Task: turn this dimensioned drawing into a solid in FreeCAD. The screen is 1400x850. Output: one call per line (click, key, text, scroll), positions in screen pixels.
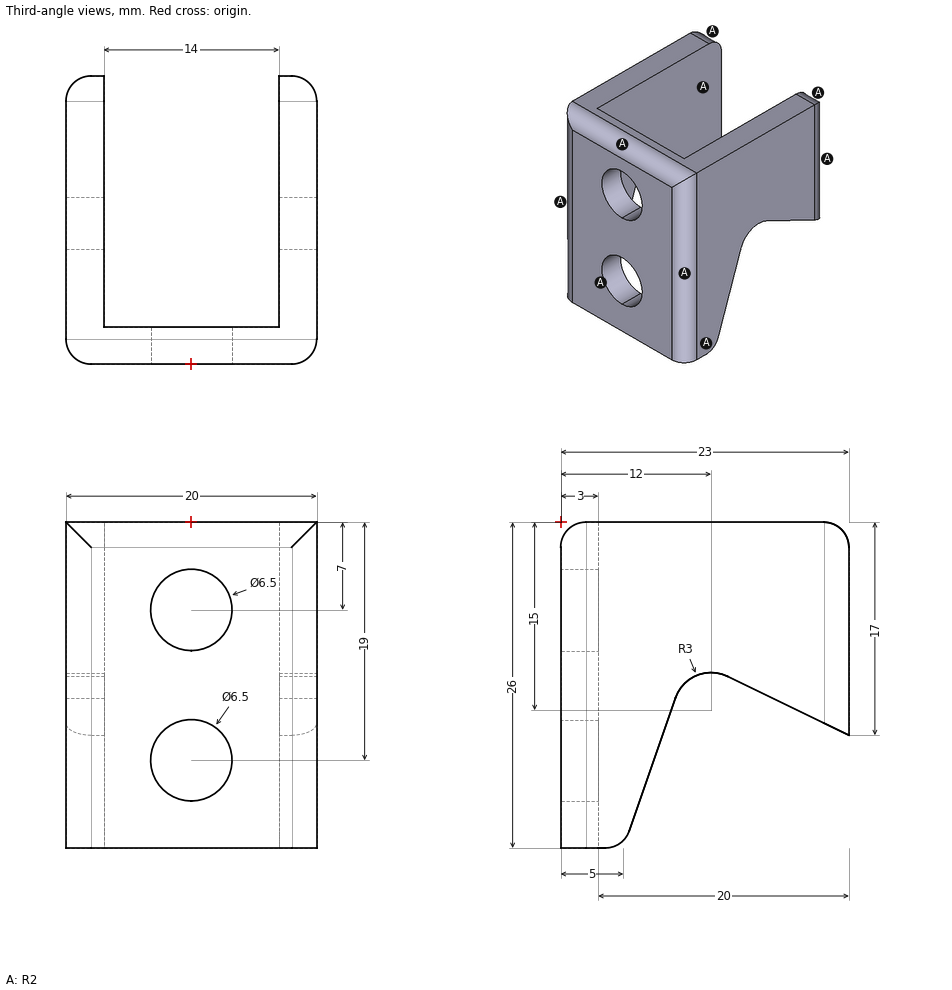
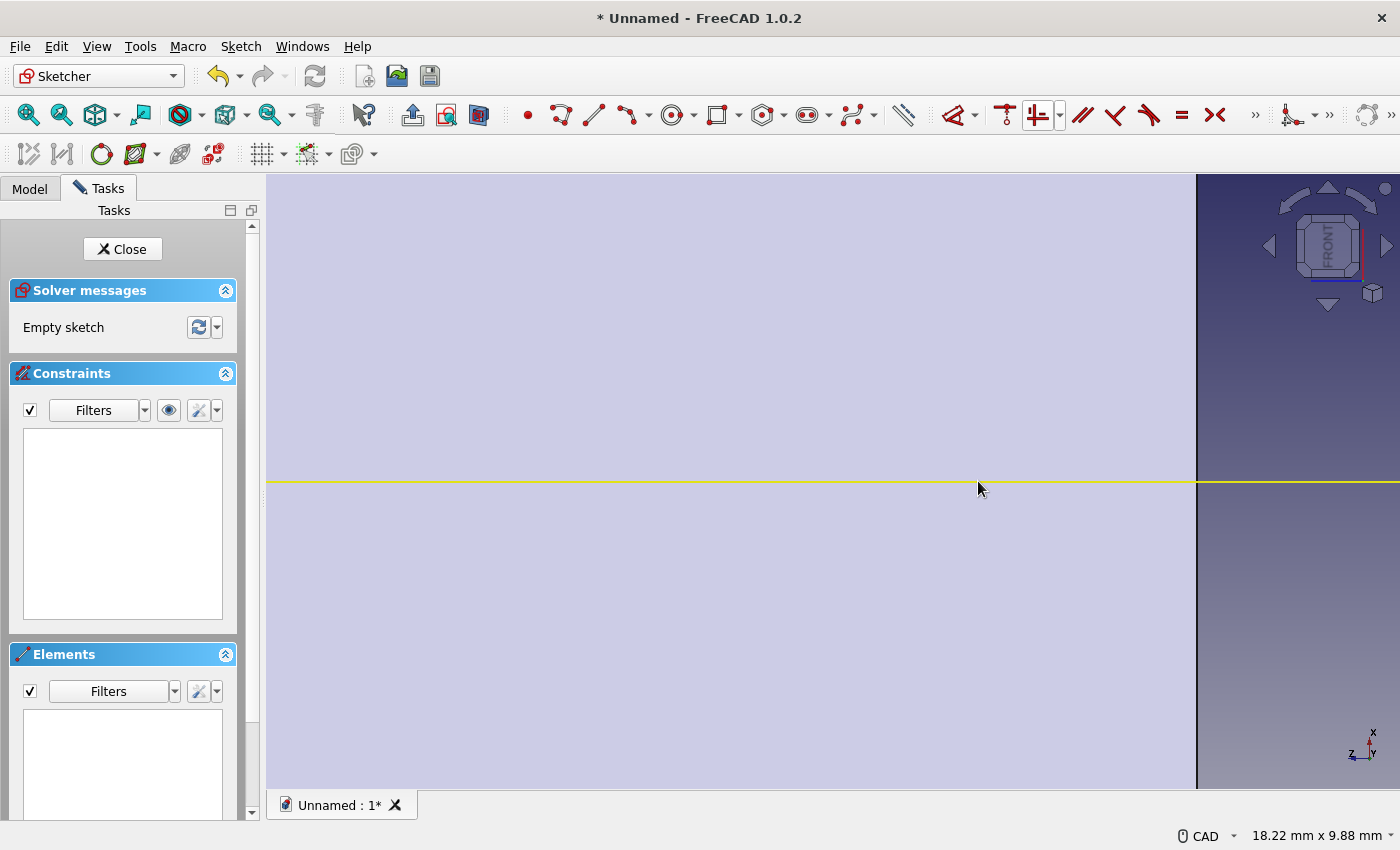
click(672, 116)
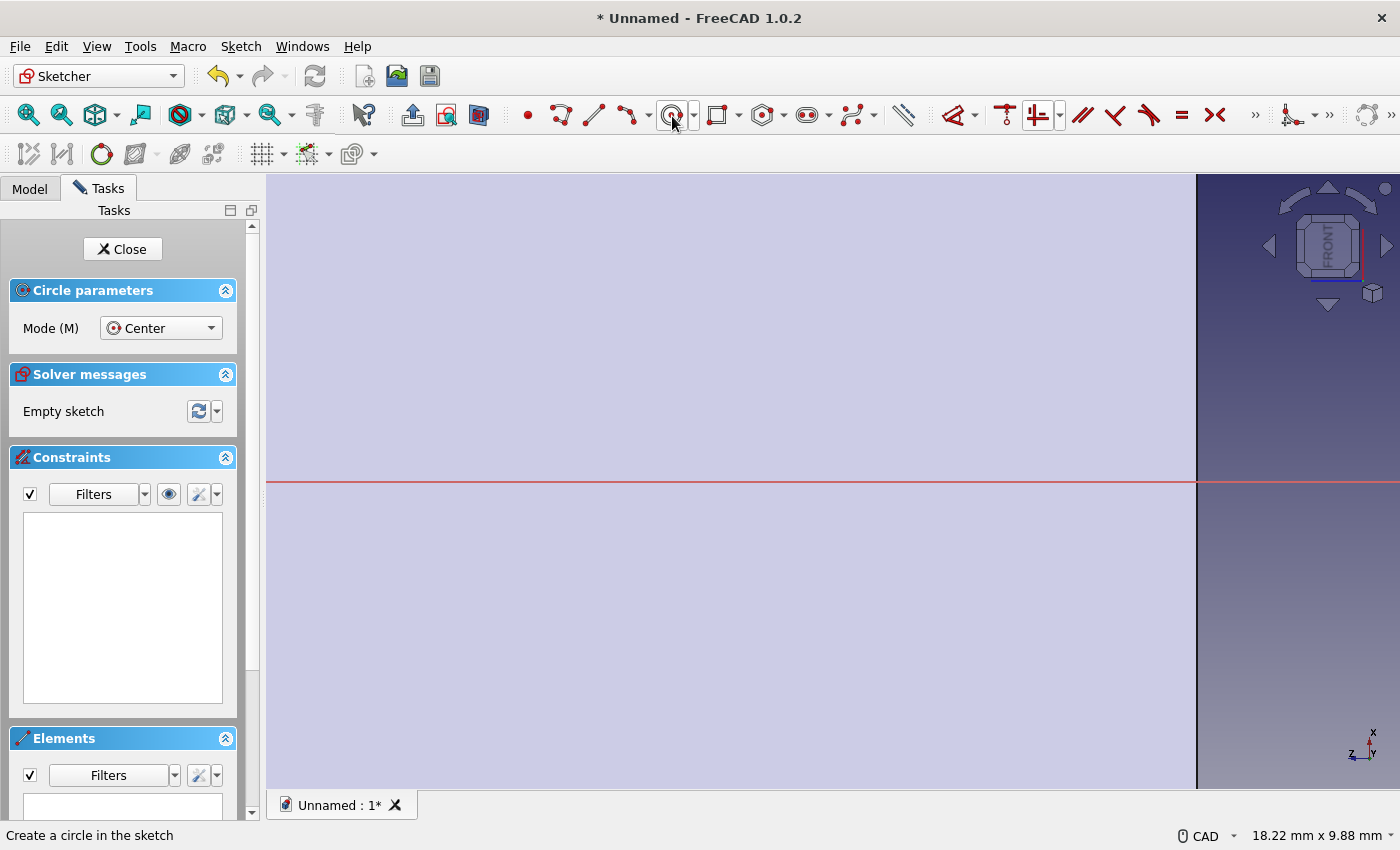
click(762, 482)
click(905, 338)
key(Escape)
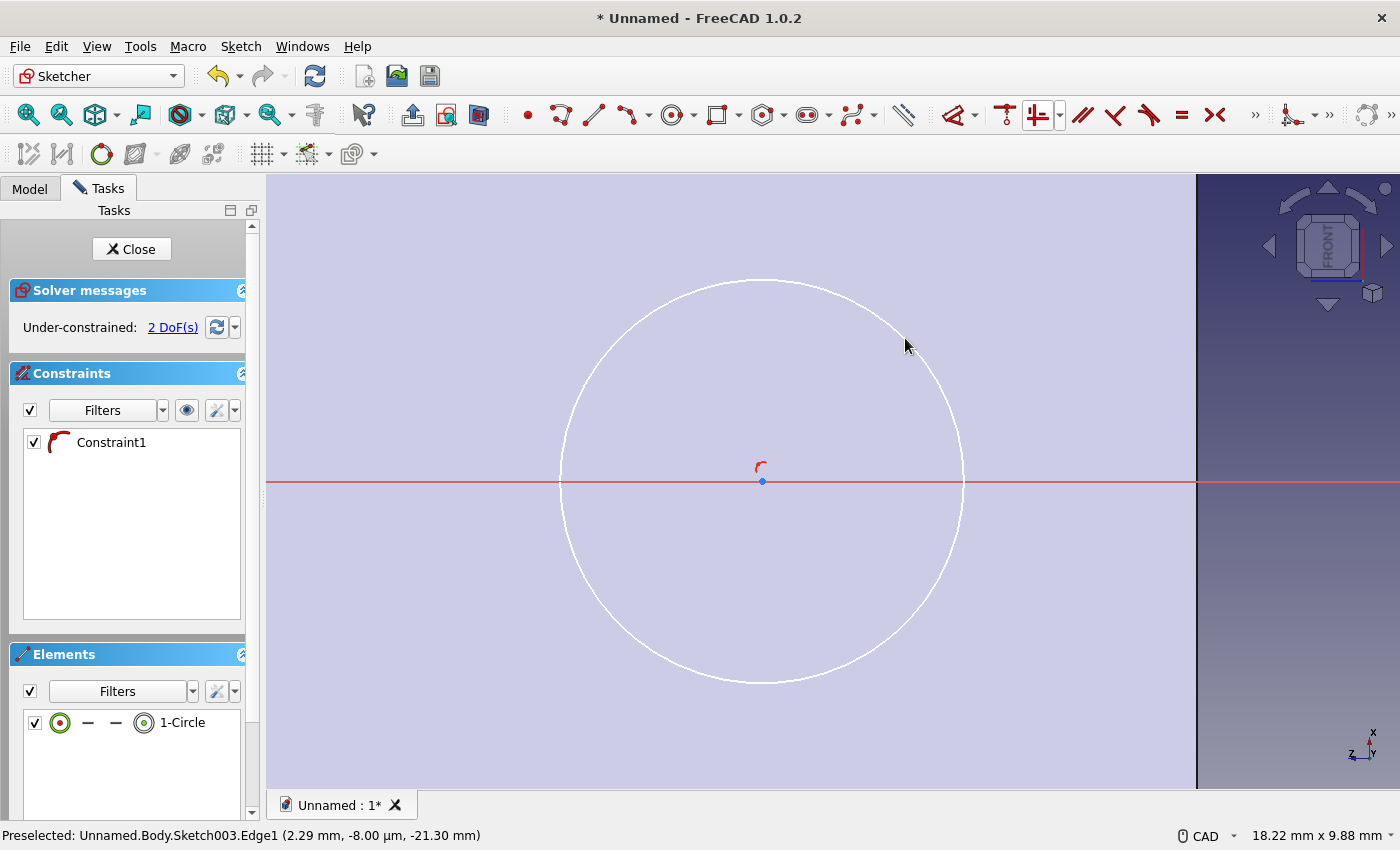
click(952, 116)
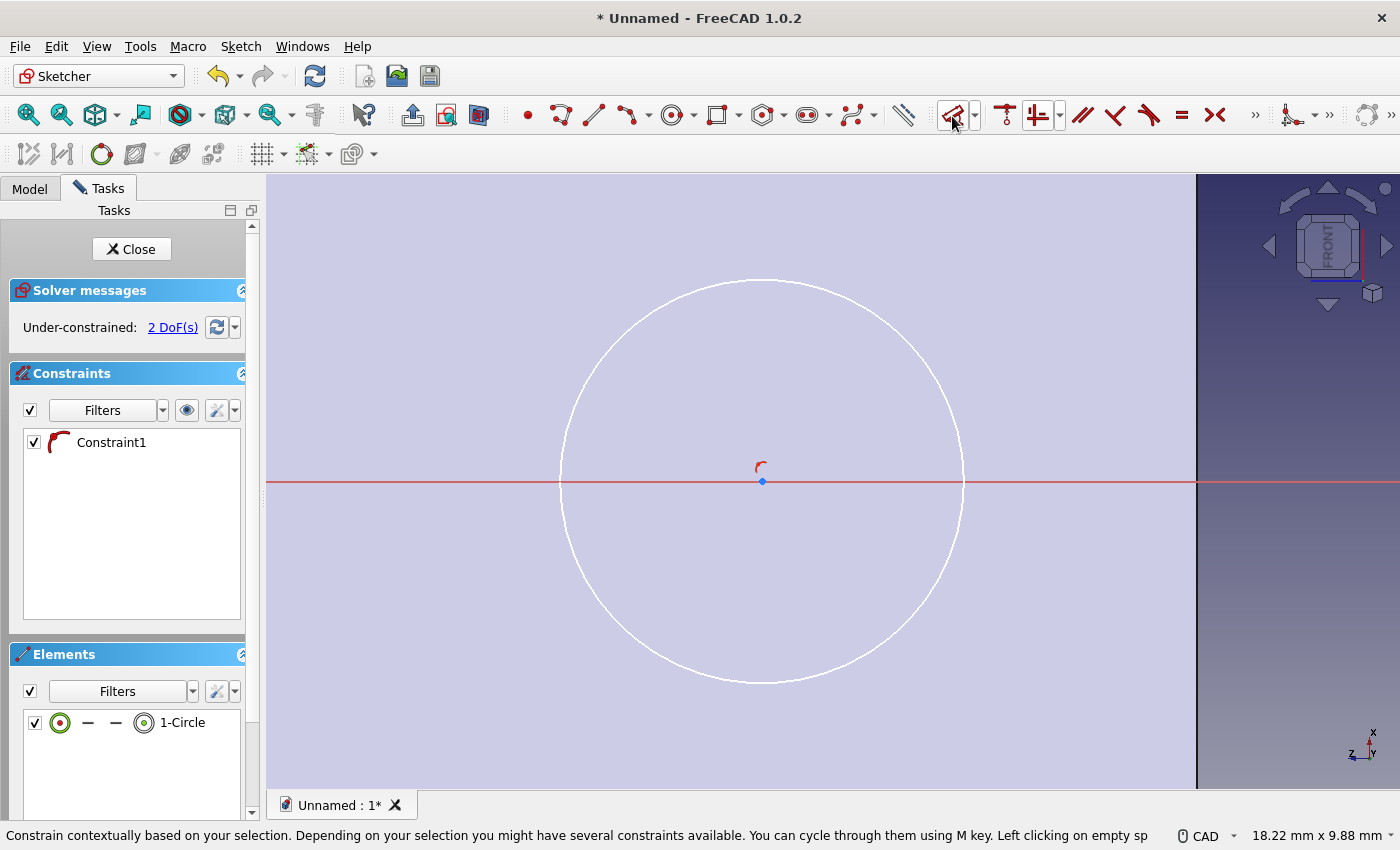
click(904, 338)
click(927, 315)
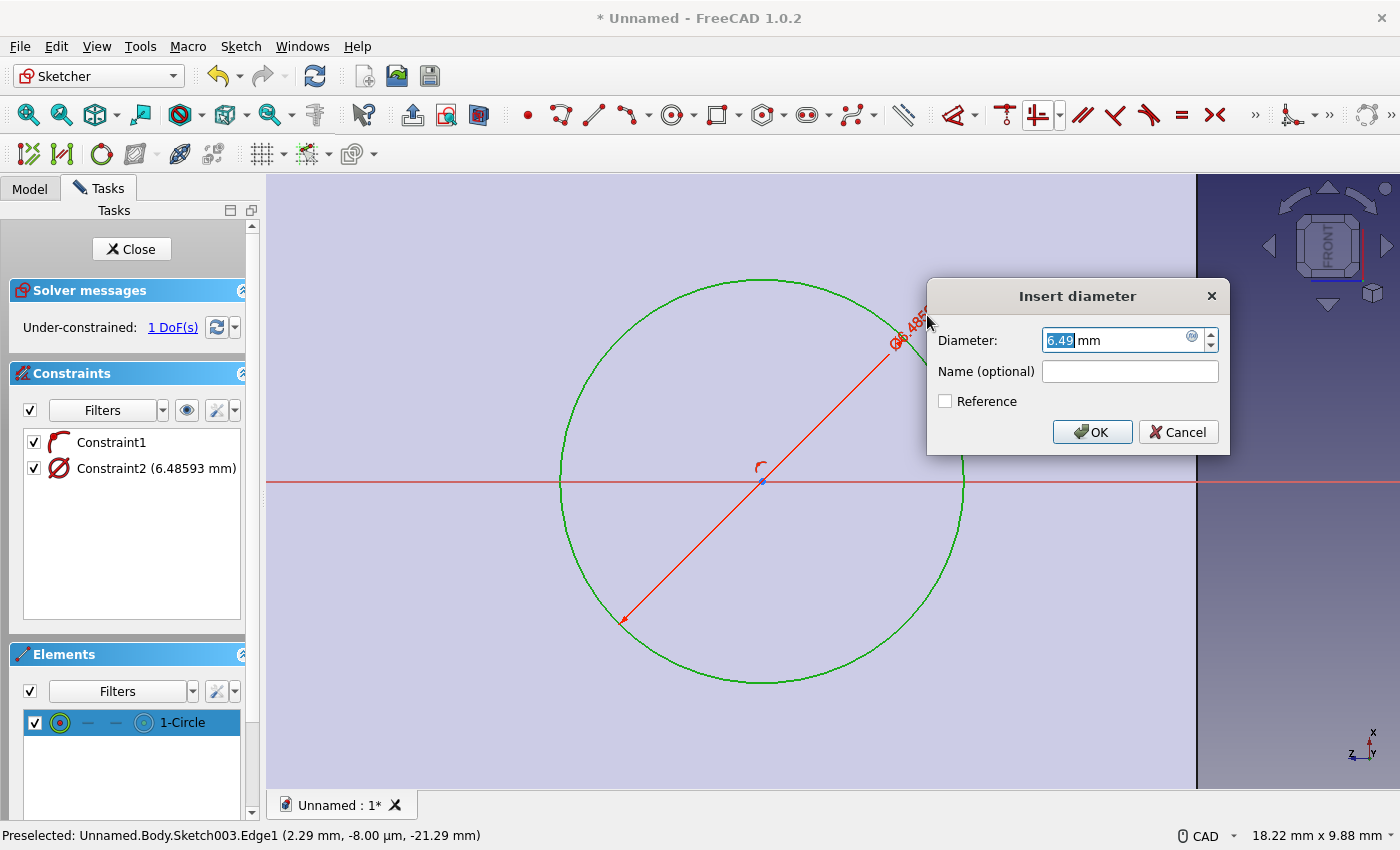
text(6.5)
key(Return)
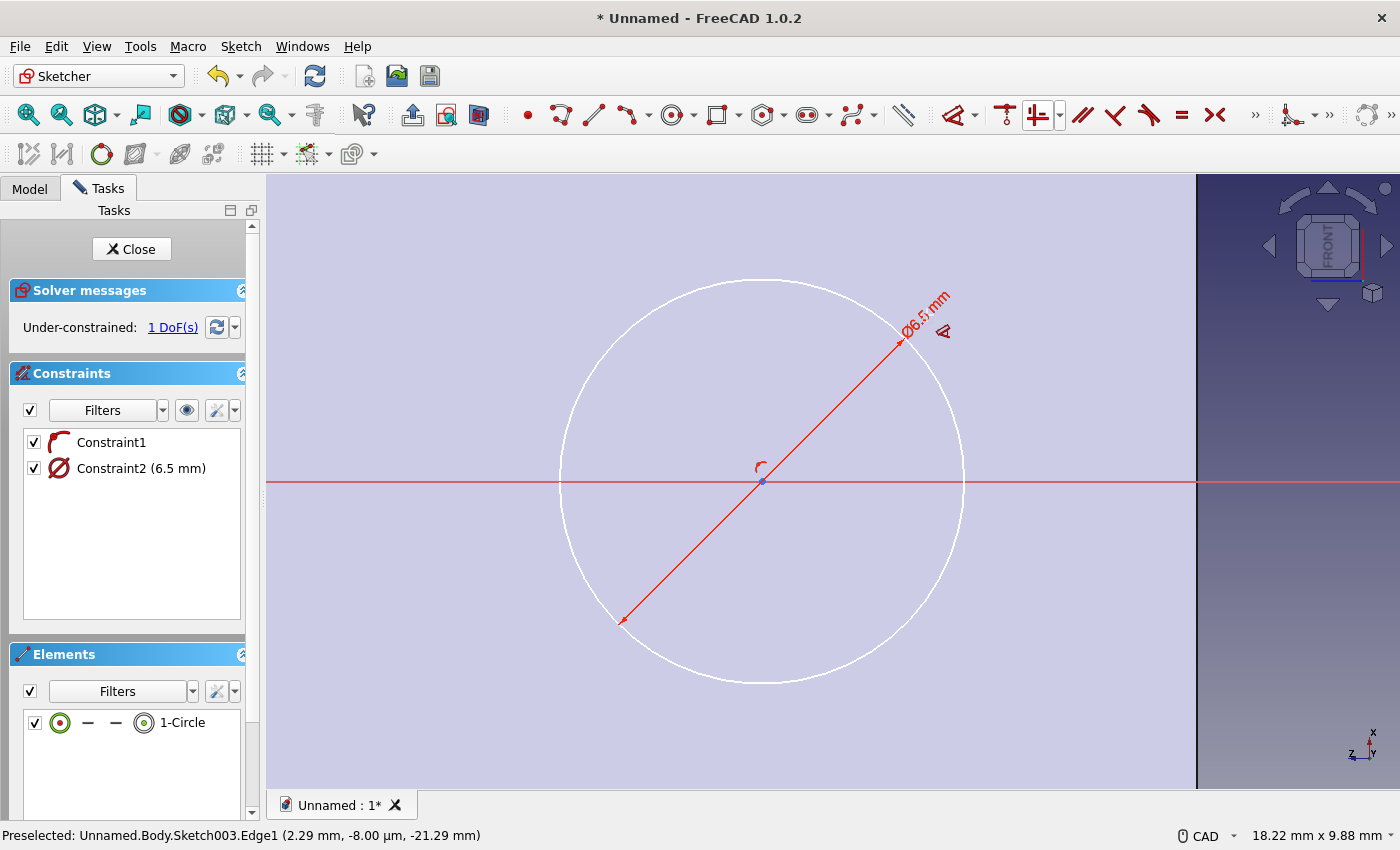
click(762, 482)
click(528, 516)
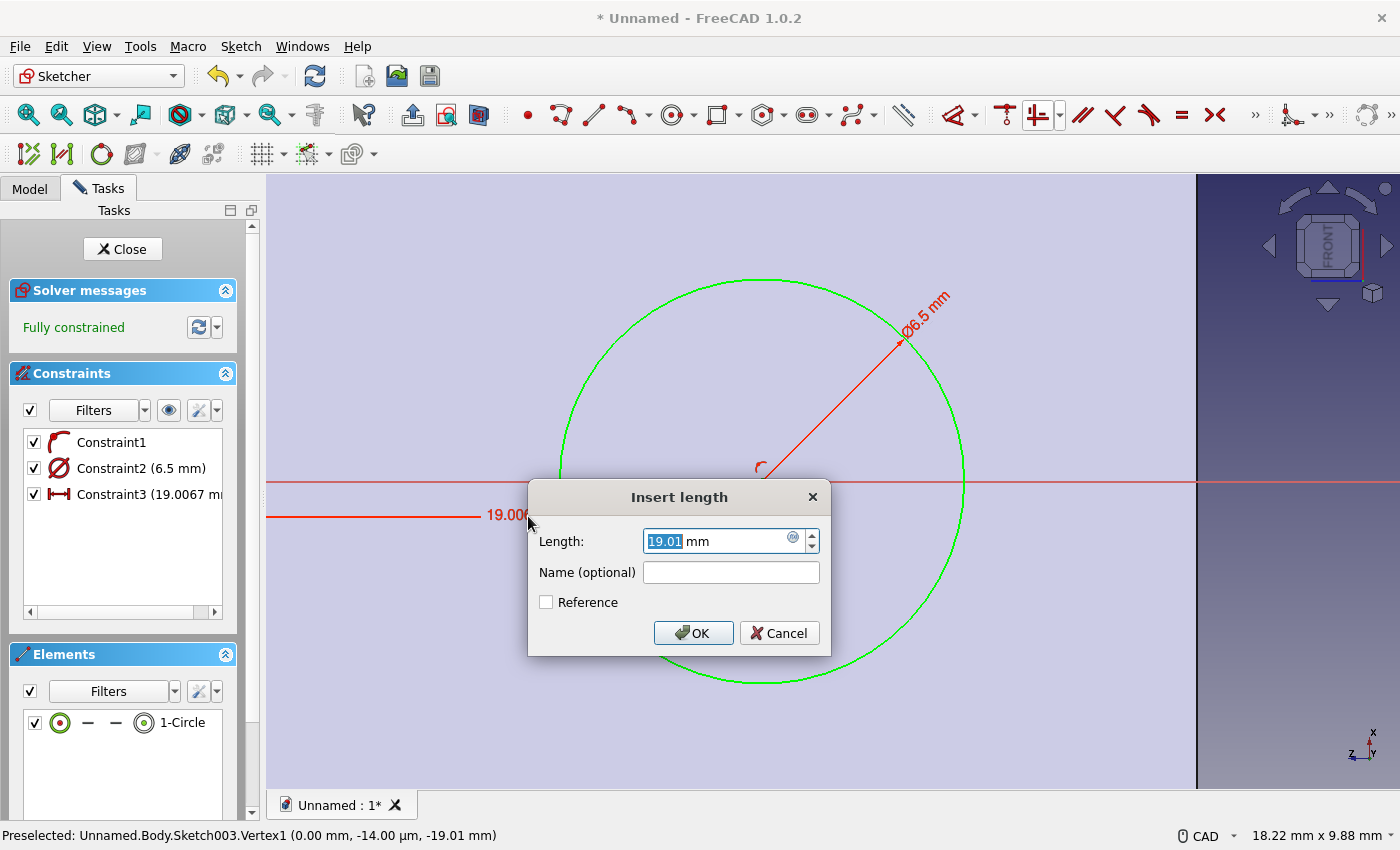
text(19)
key(Return)
key(Escape)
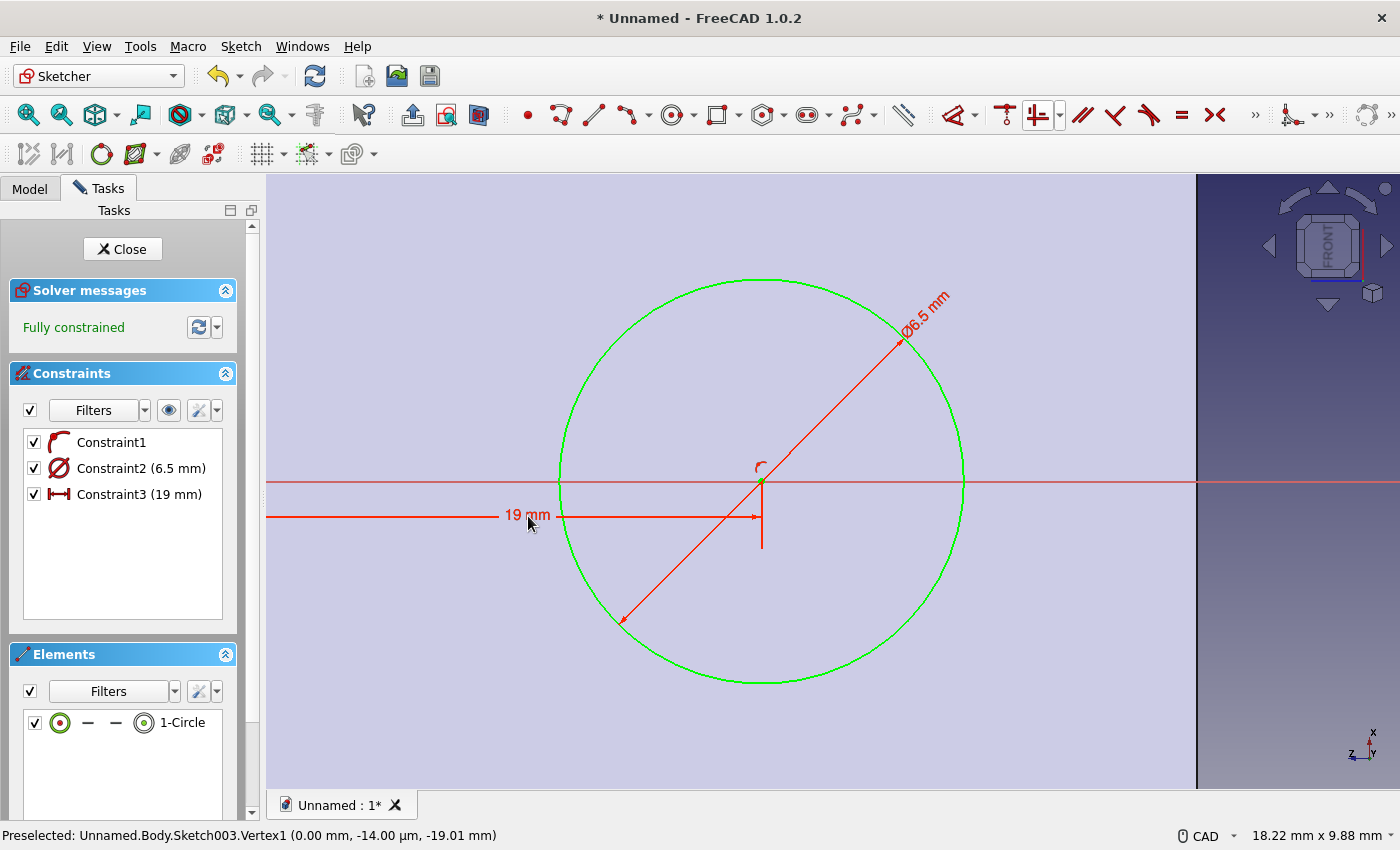
click(123, 249)